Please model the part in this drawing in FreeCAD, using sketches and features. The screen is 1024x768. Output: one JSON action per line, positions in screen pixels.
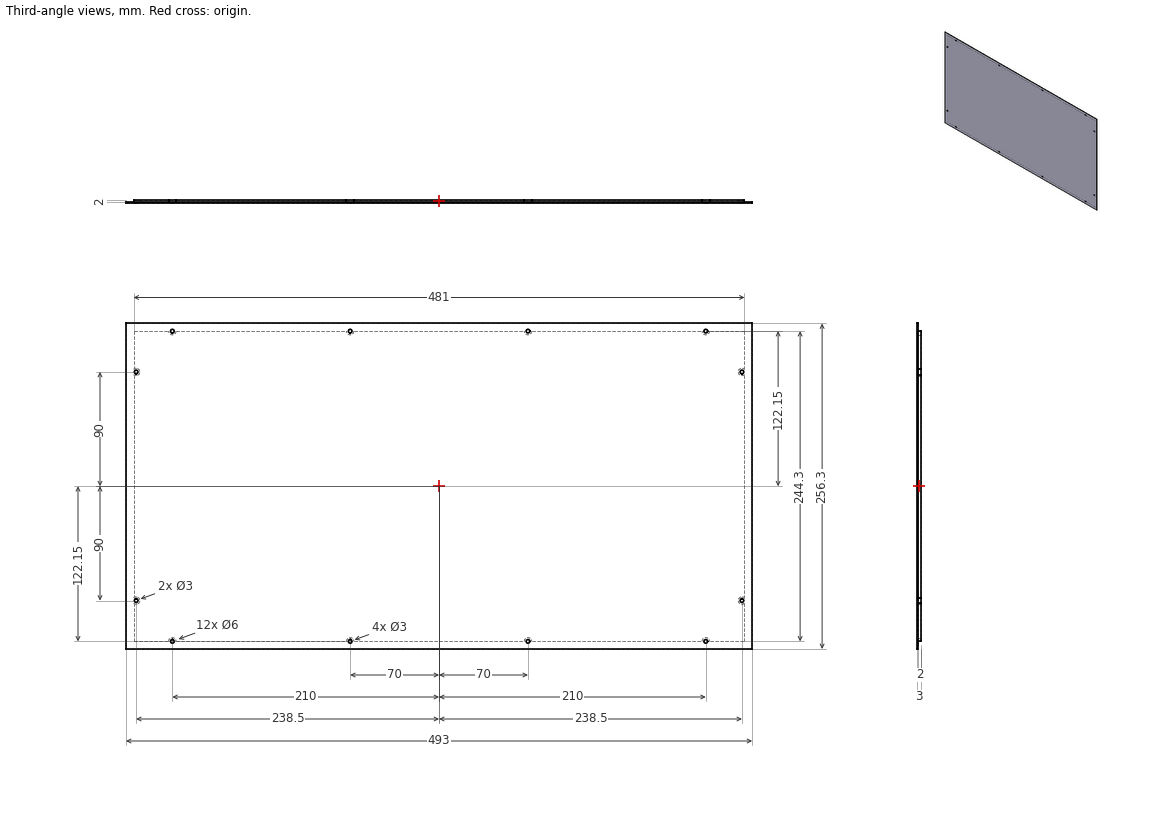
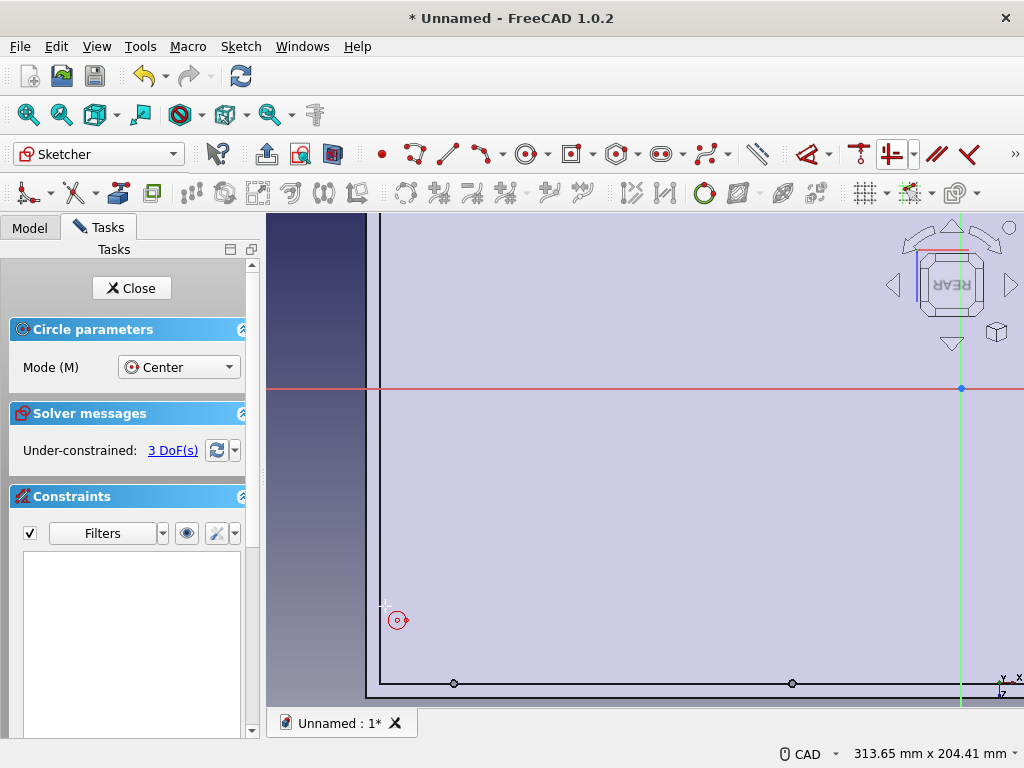
{"action": "left_click", "coordinate": [385, 606]}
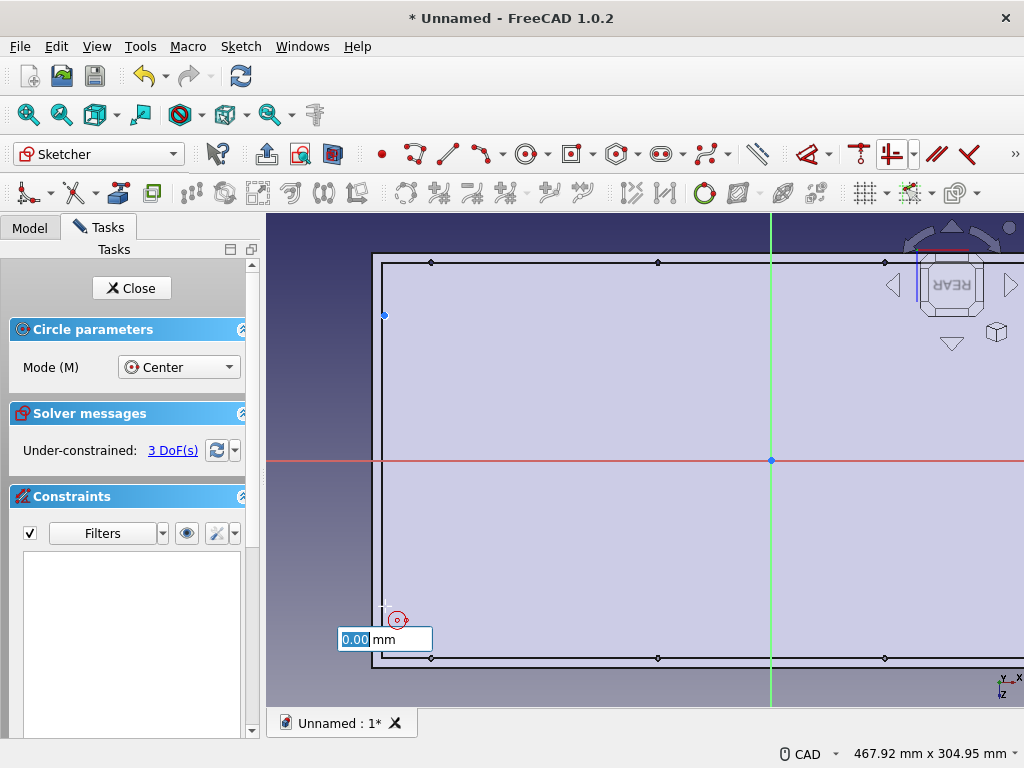
{"action": "scroll", "coordinate": [387, 605], "scroll_direction": "up", "scroll_amount": 10}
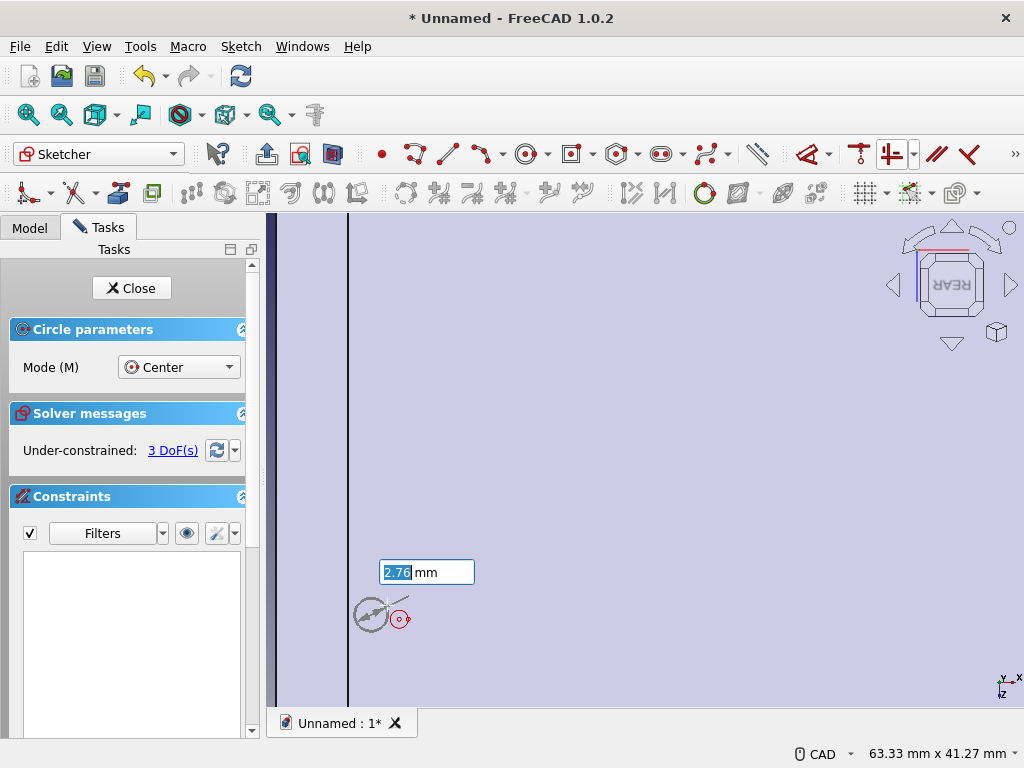
{"action": "left_click", "coordinate": [385, 597]}
{"action": "key", "text": "Escape"}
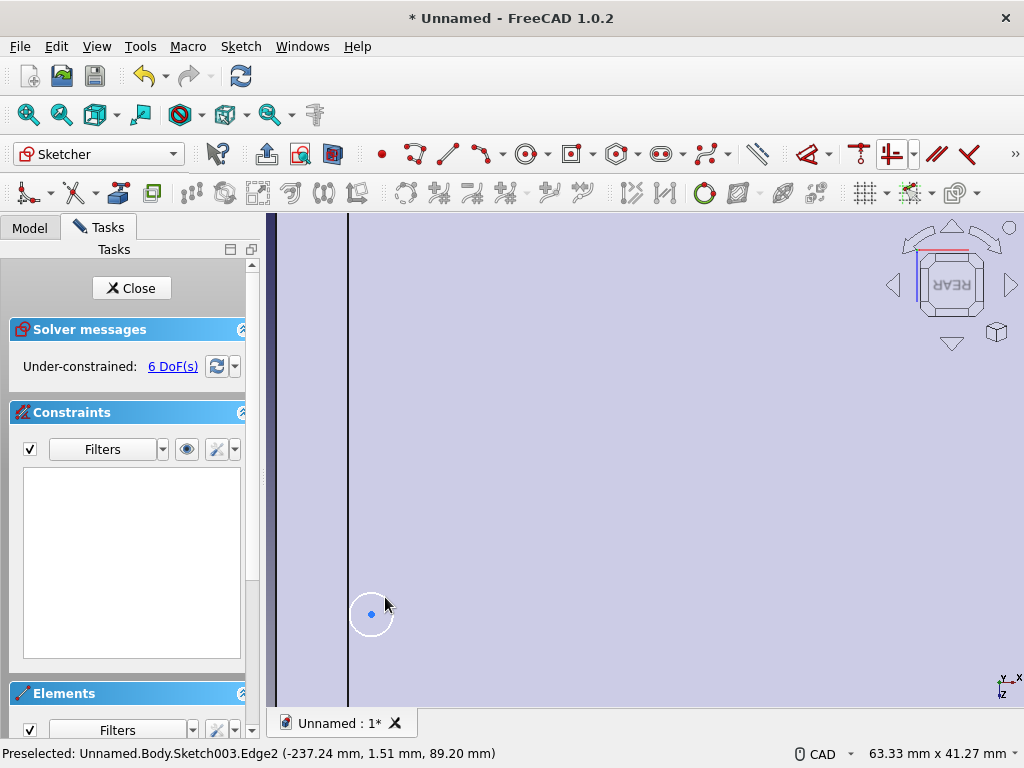
{"action": "scroll", "coordinate": [387, 605], "scroll_direction": "down", "scroll_amount": 10}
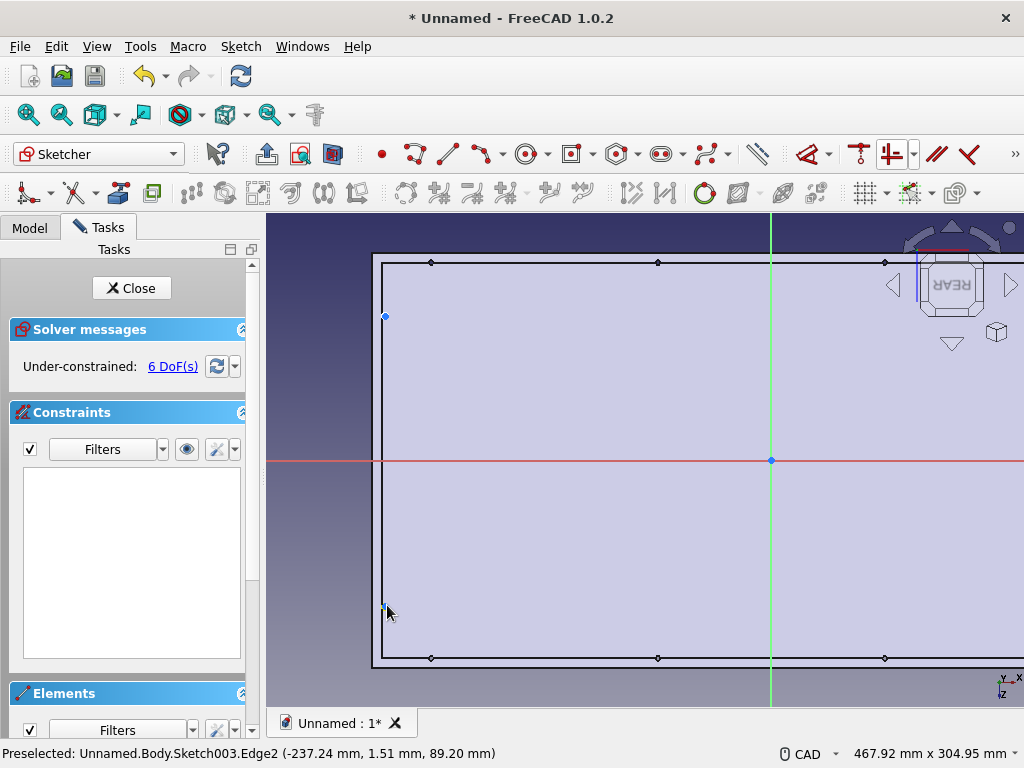
{"action": "scroll", "coordinate": [387, 314], "scroll_direction": "up", "scroll_amount": 8}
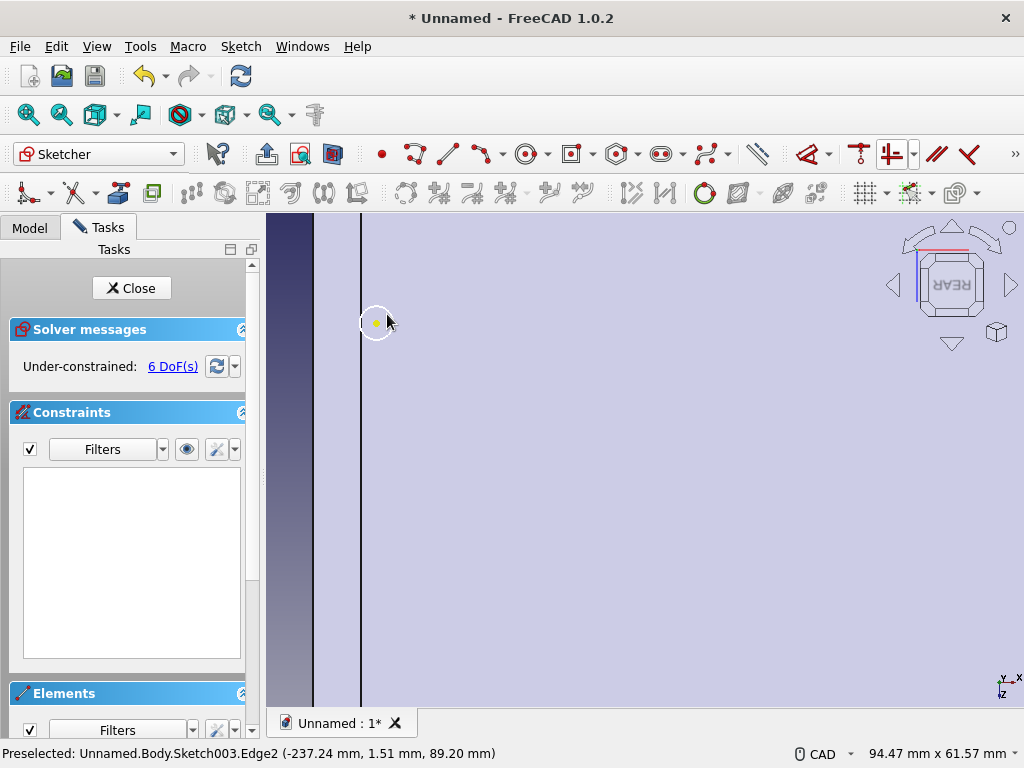
{"action": "left_click", "coordinate": [388, 311]}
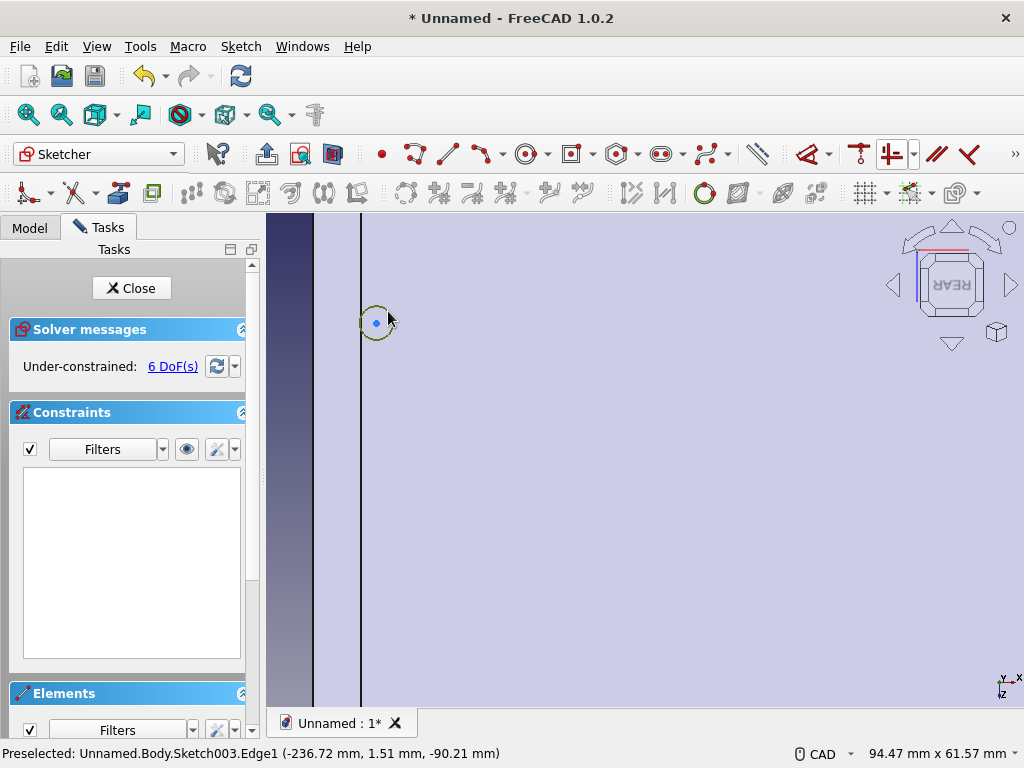
{"action": "scroll", "coordinate": [386, 314], "scroll_direction": "down", "scroll_amount": 8}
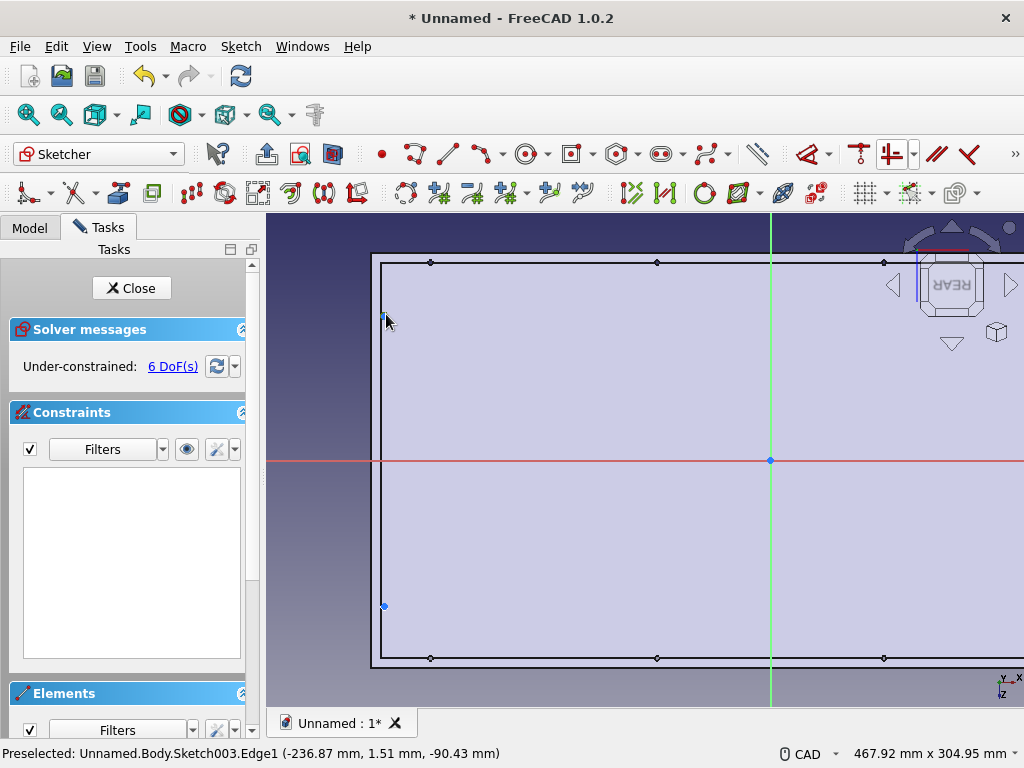
{"action": "scroll", "coordinate": [386, 605], "scroll_direction": "up", "scroll_amount": 8}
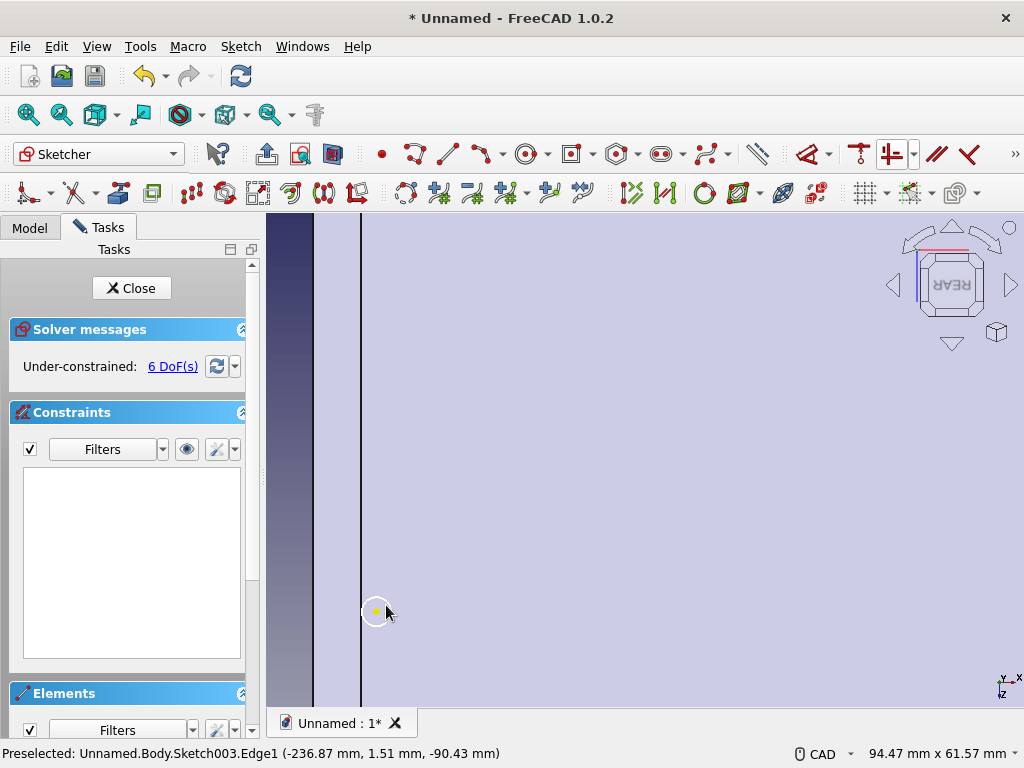
{"action": "left_click", "coordinate": [387, 601]}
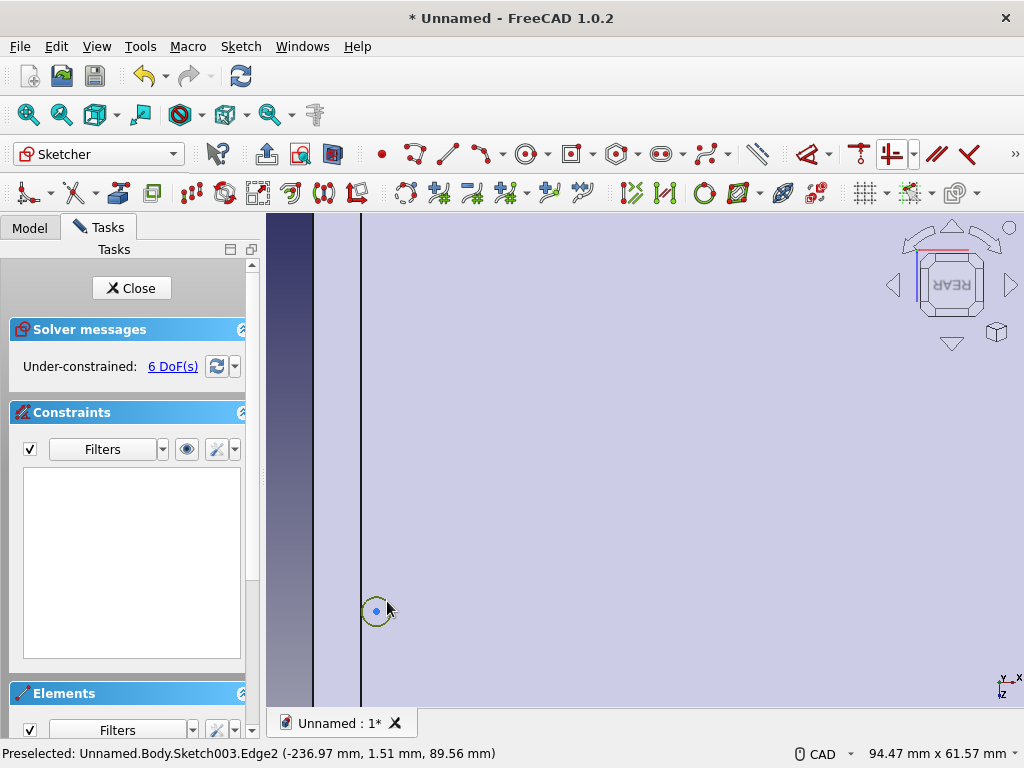
{"action": "key", "text": "e"}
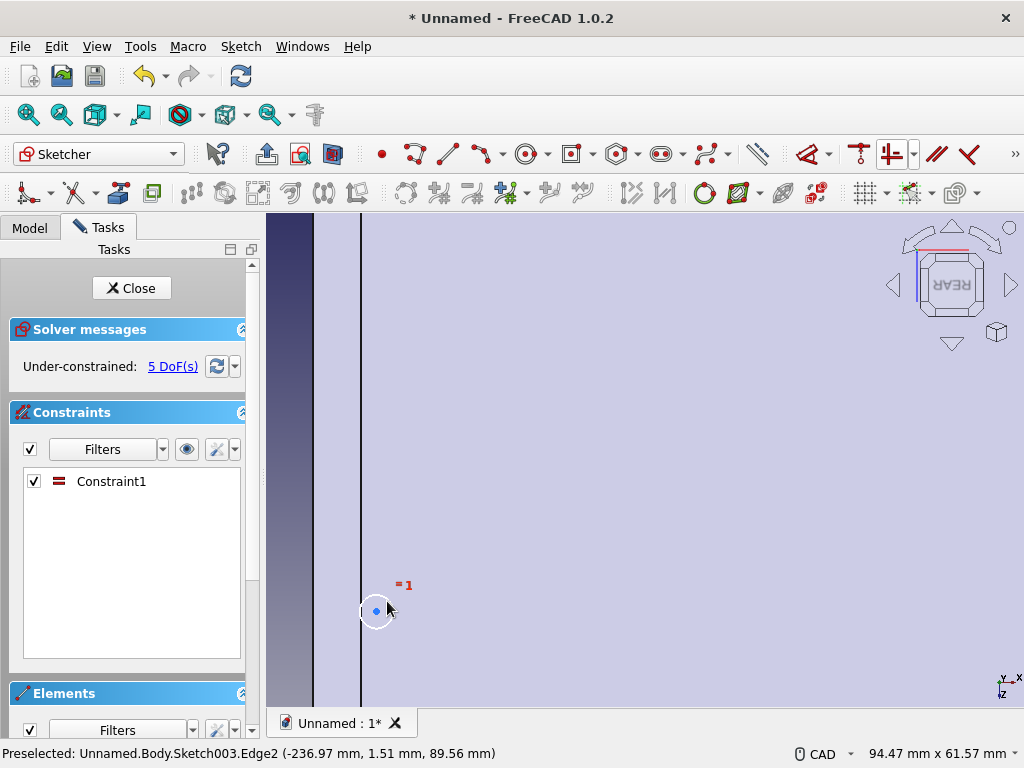
{"action": "scroll", "coordinate": [386, 605], "scroll_direction": "down", "scroll_amount": 8}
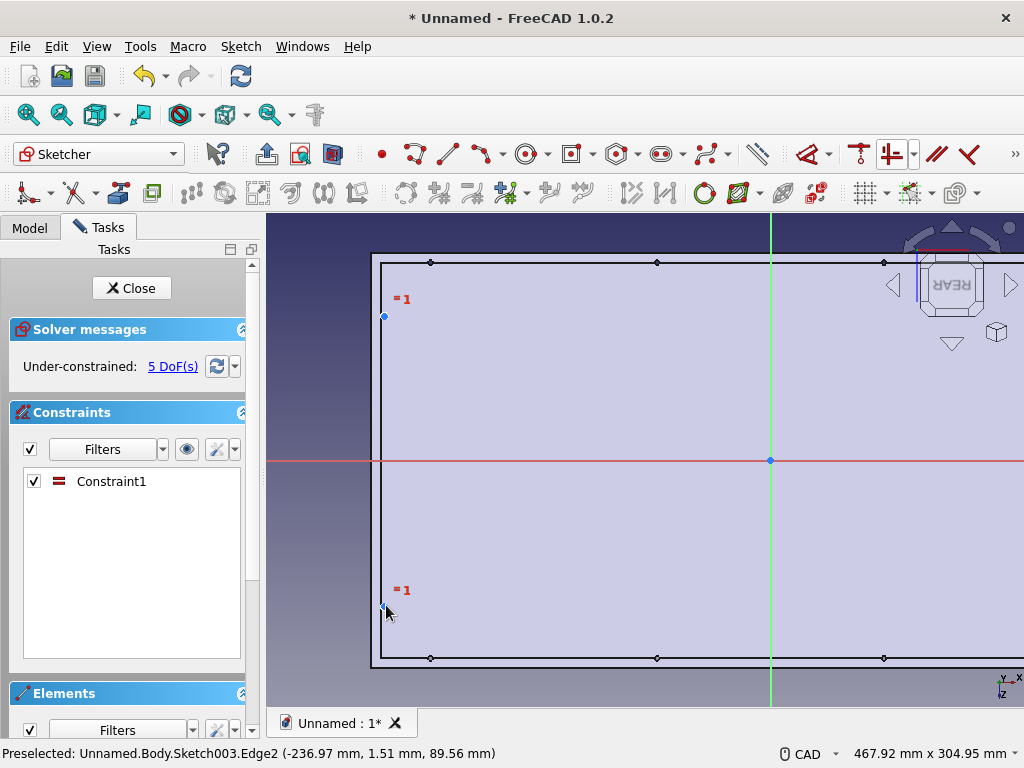
{"action": "left_click", "coordinate": [384, 316]}